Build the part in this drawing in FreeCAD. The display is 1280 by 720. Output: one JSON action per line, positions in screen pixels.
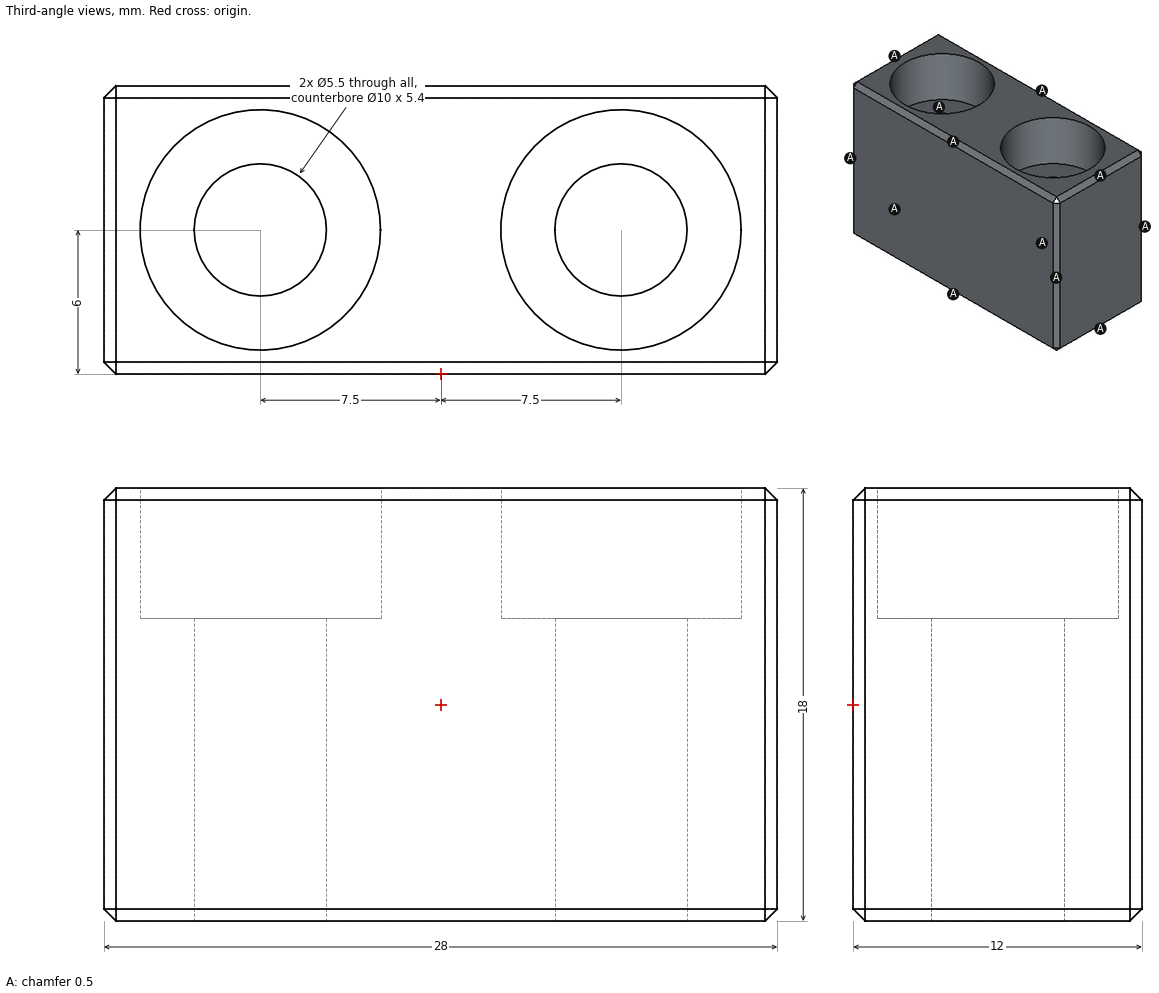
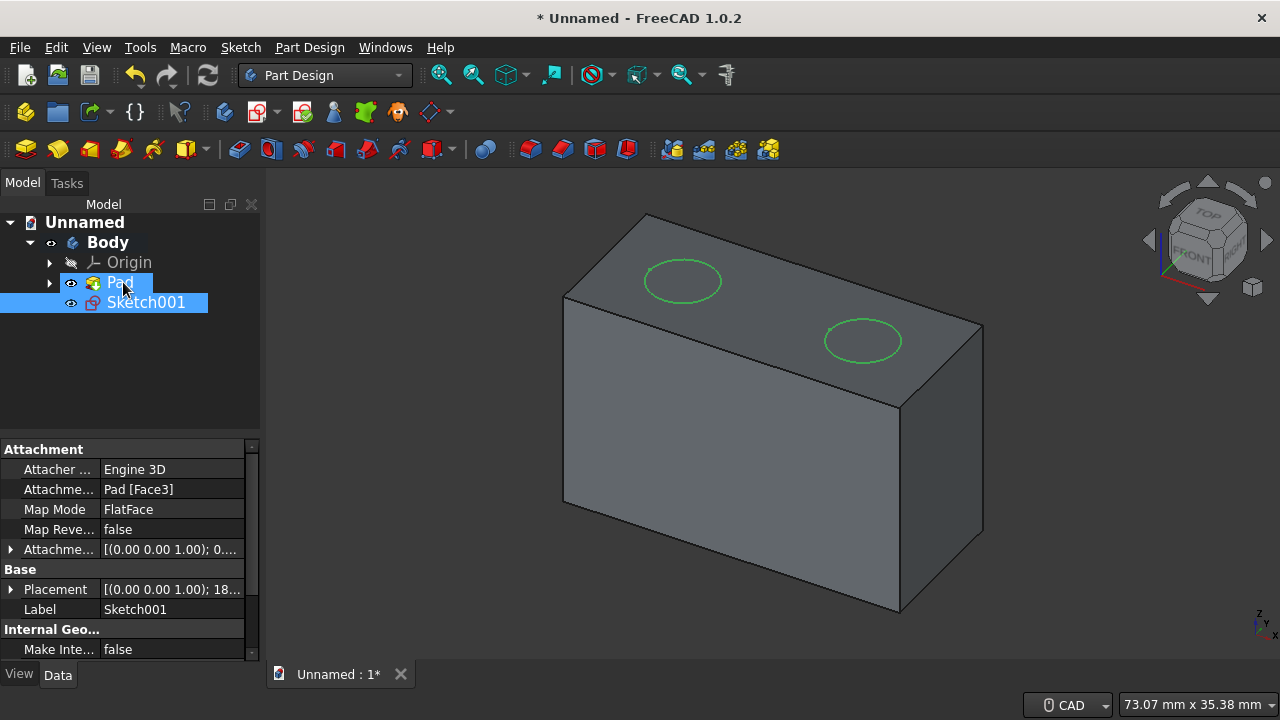
{"action": "left_click", "coordinate": [272, 150]}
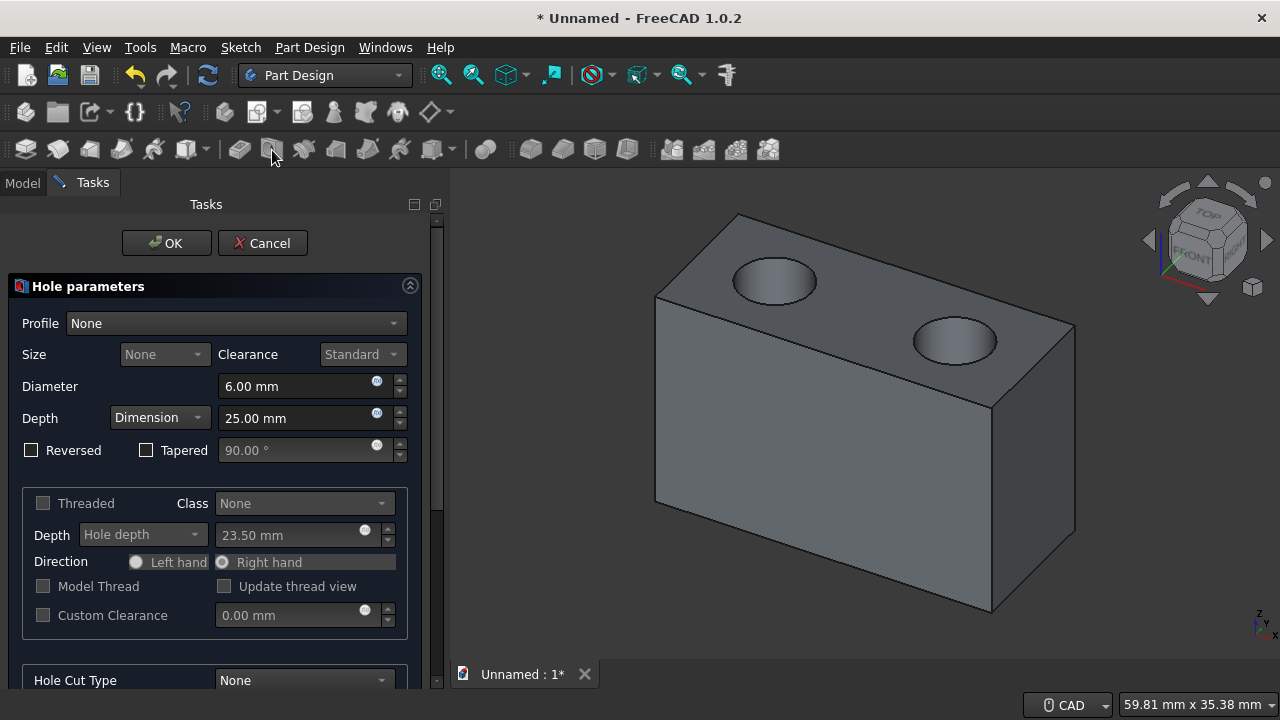
{"action": "triple_click", "coordinate": [305, 386]}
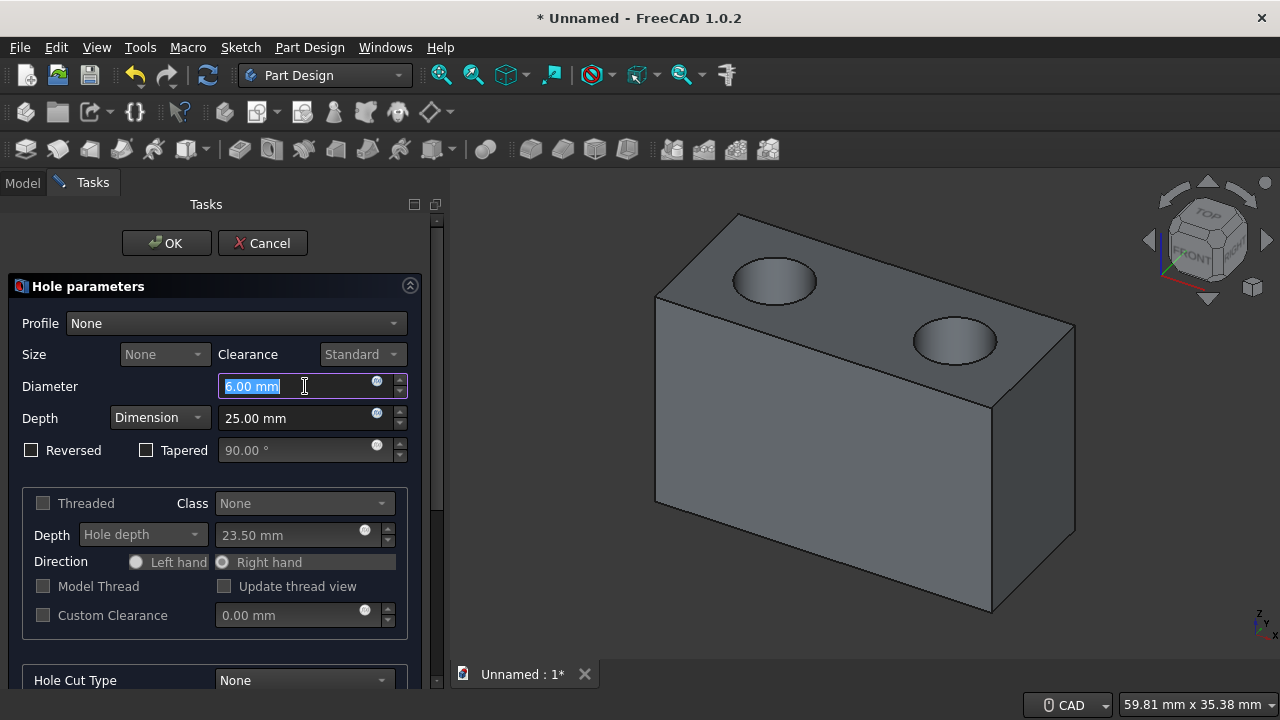
{"action": "type", "text": "5.5"}
{"action": "key", "text": "Tab"}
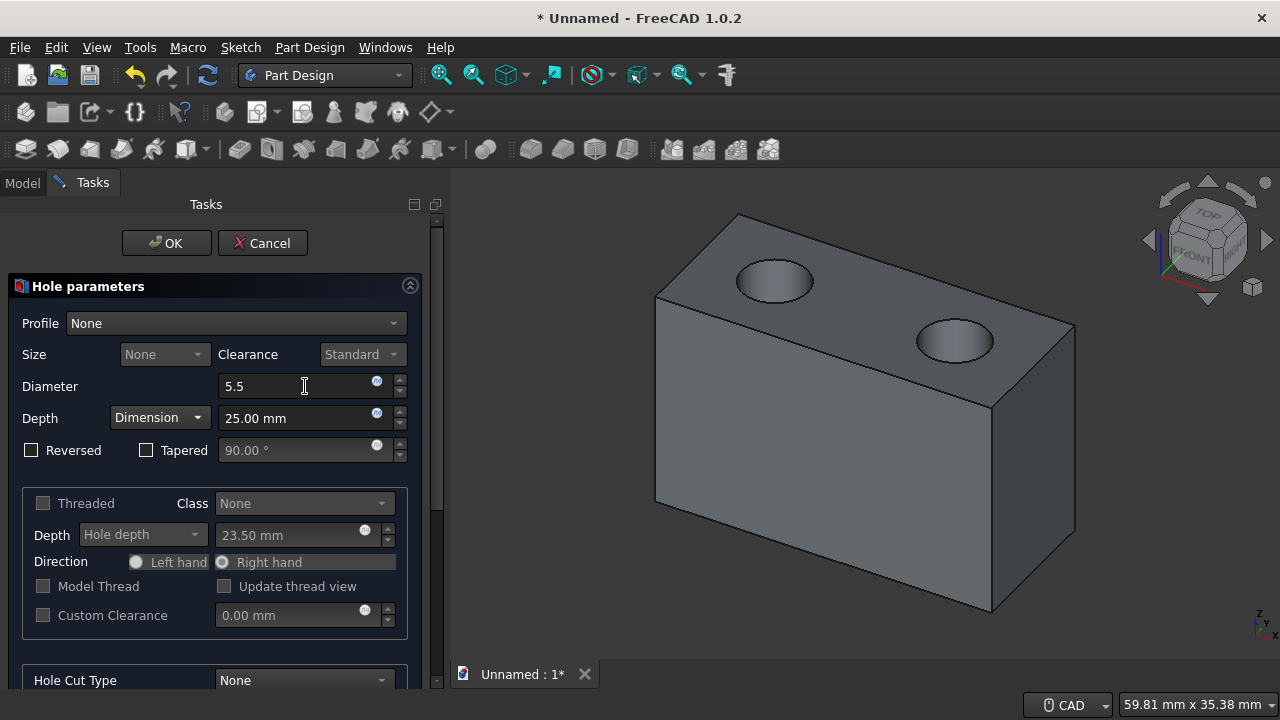
{"action": "left_click", "coordinate": [161, 418]}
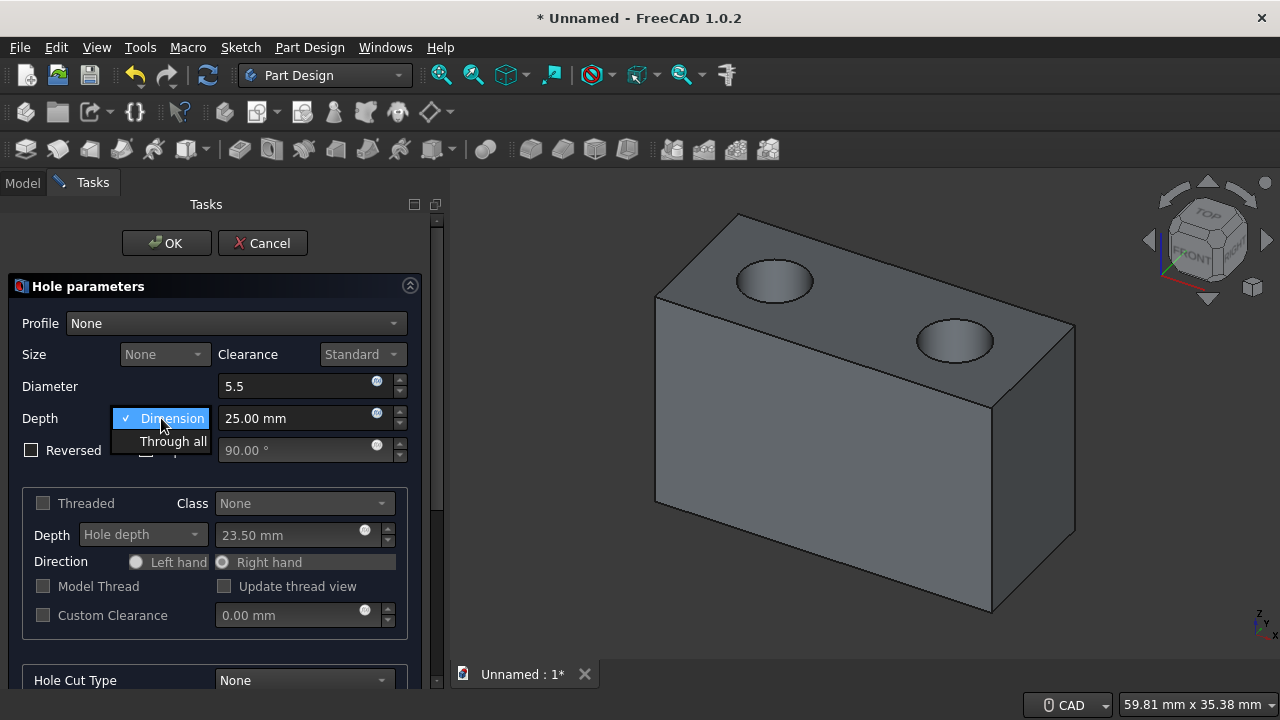
{"action": "left_click", "coordinate": [160, 442]}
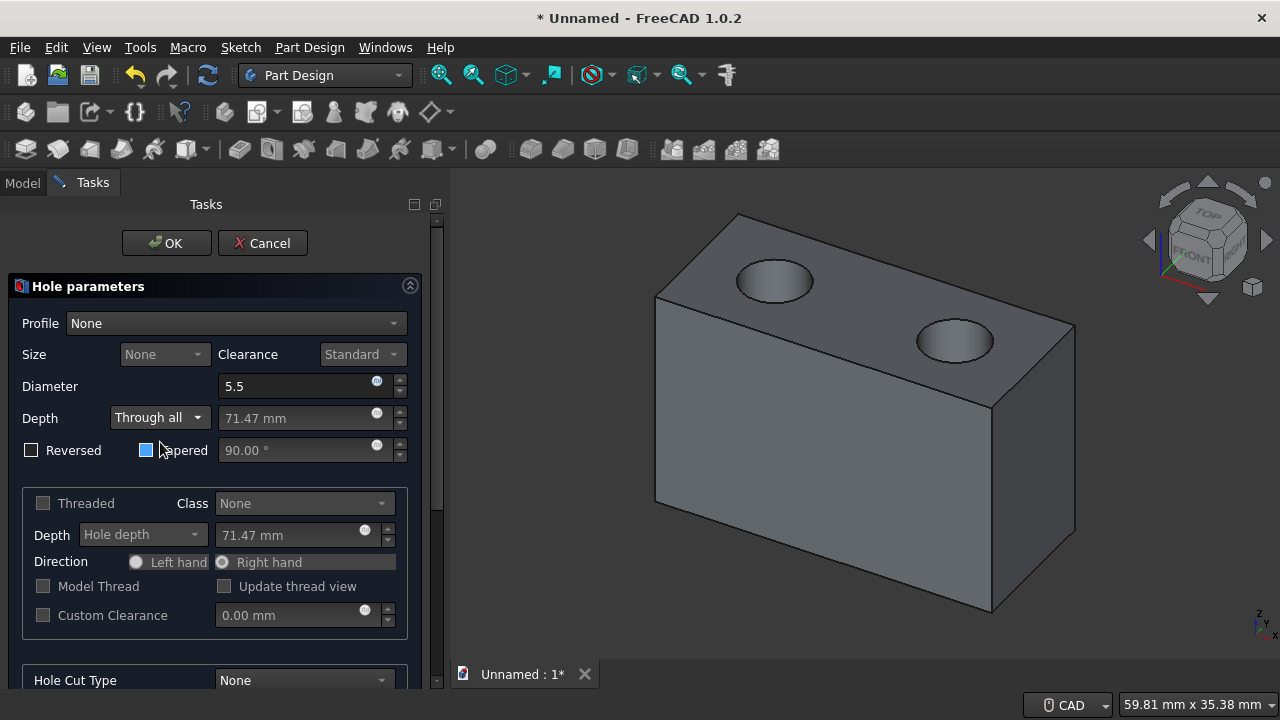
{"action": "scroll", "coordinate": [437, 451], "scroll_direction": "down", "scroll_amount": 2}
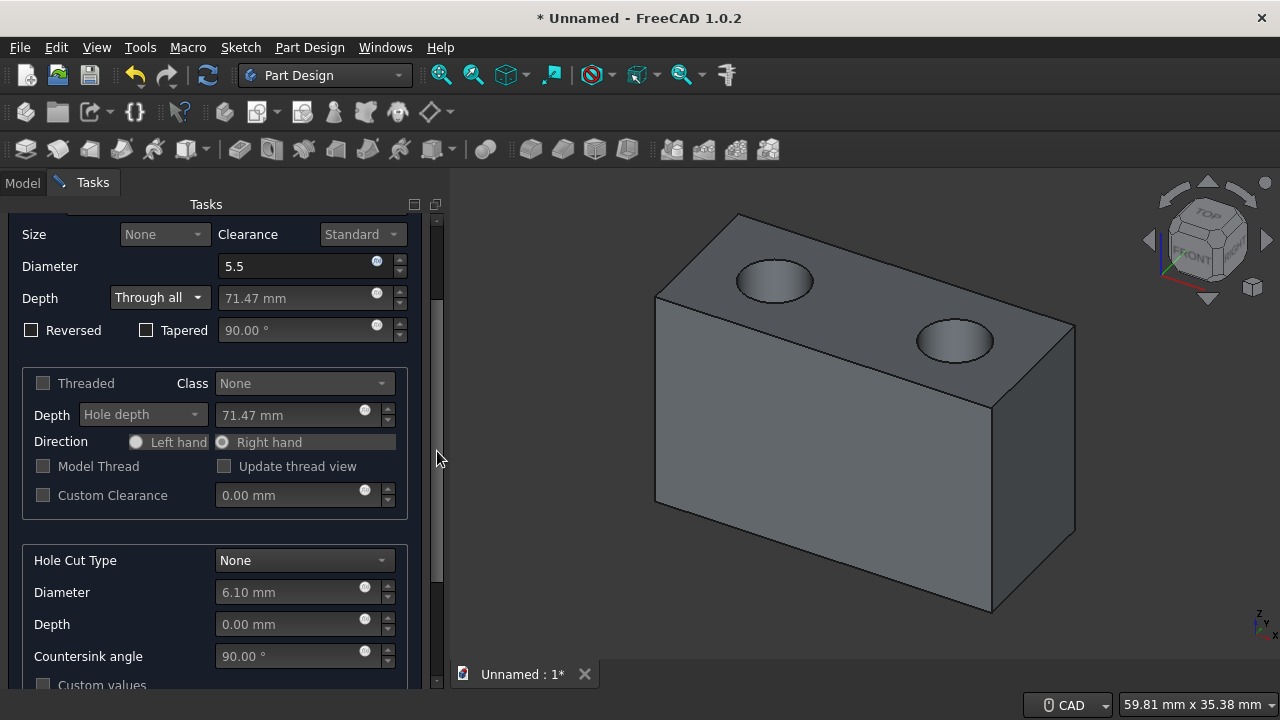
{"action": "left_click", "coordinate": [306, 560]}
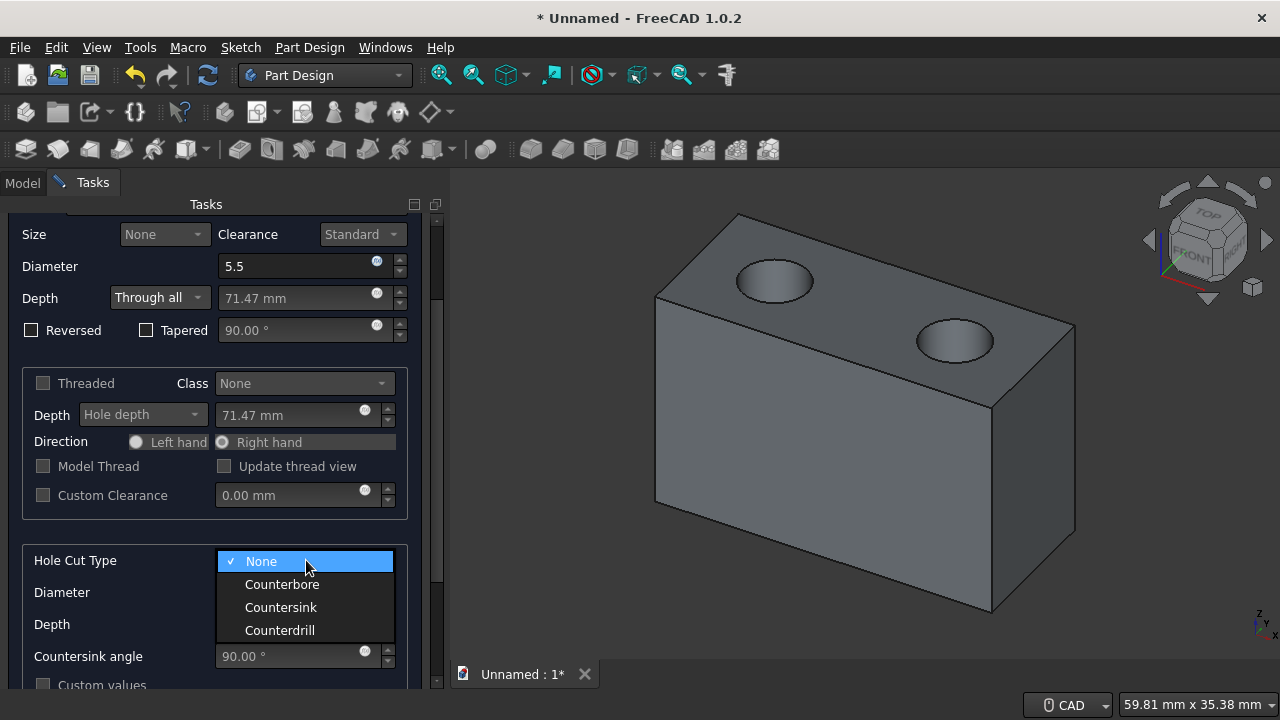
{"action": "left_click", "coordinate": [304, 584]}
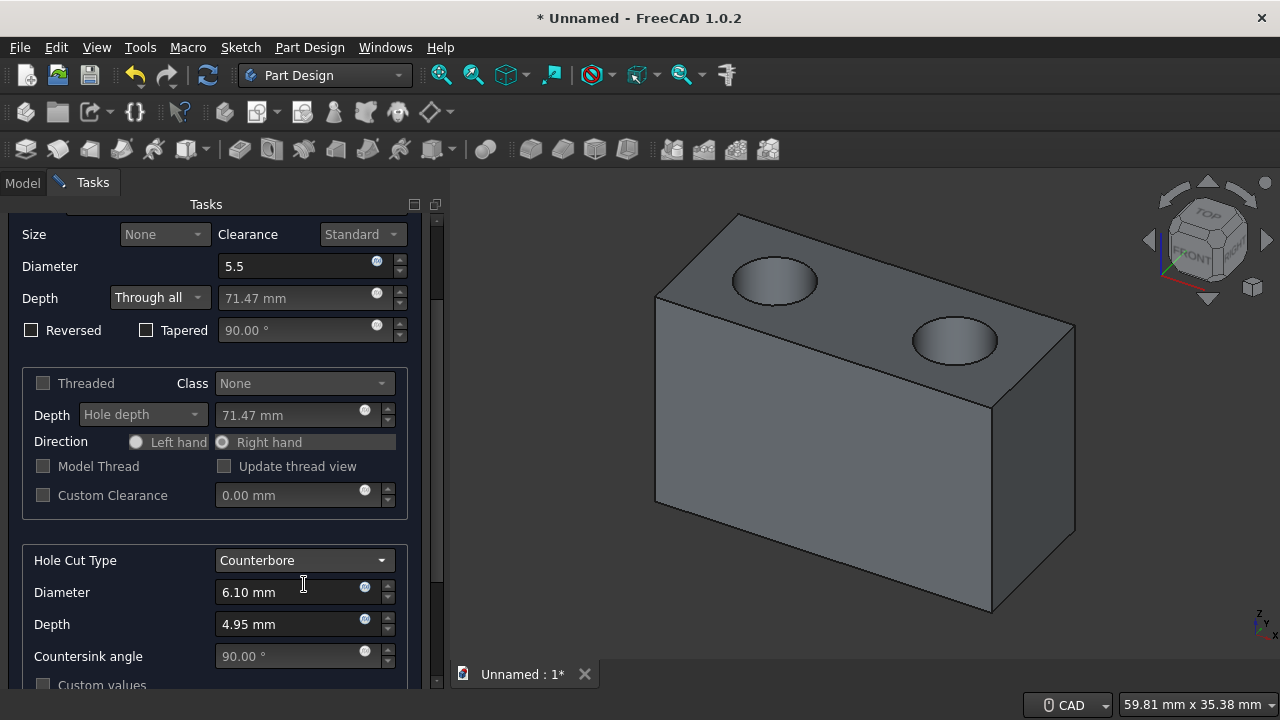
{"action": "triple_click", "coordinate": [298, 592]}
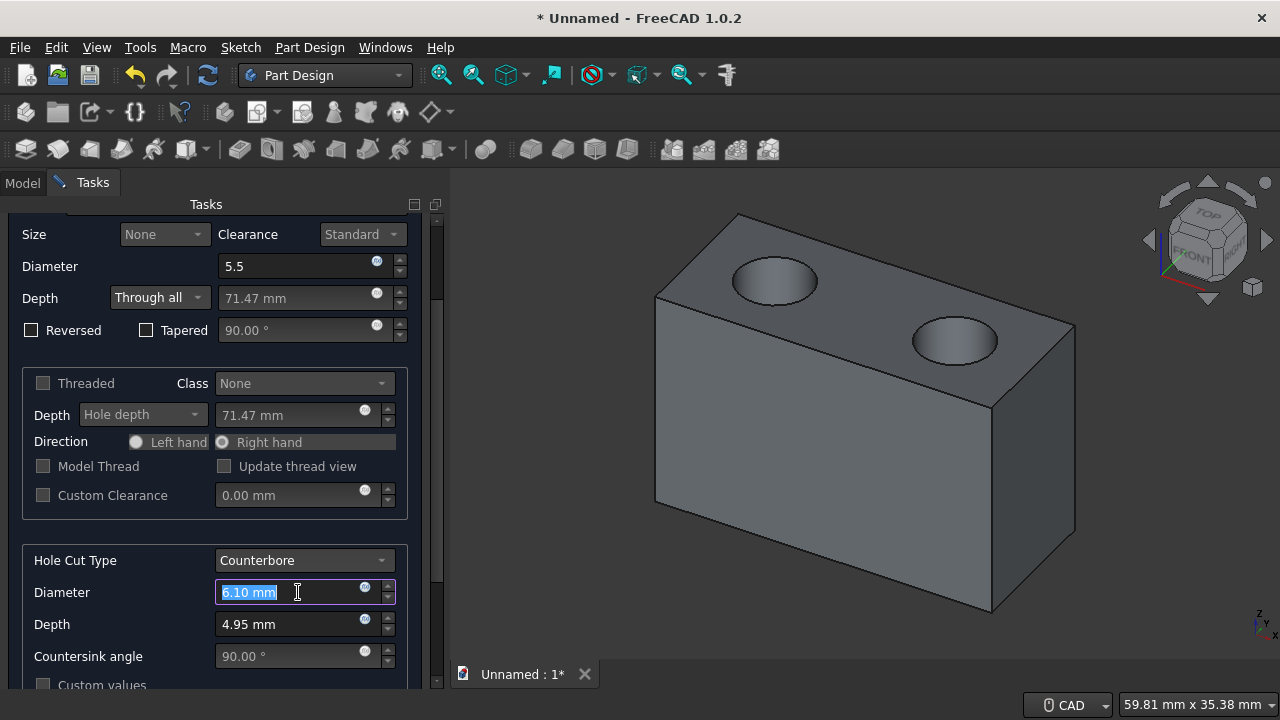
{"action": "type", "text": "10"}
{"action": "key", "text": "Tab"}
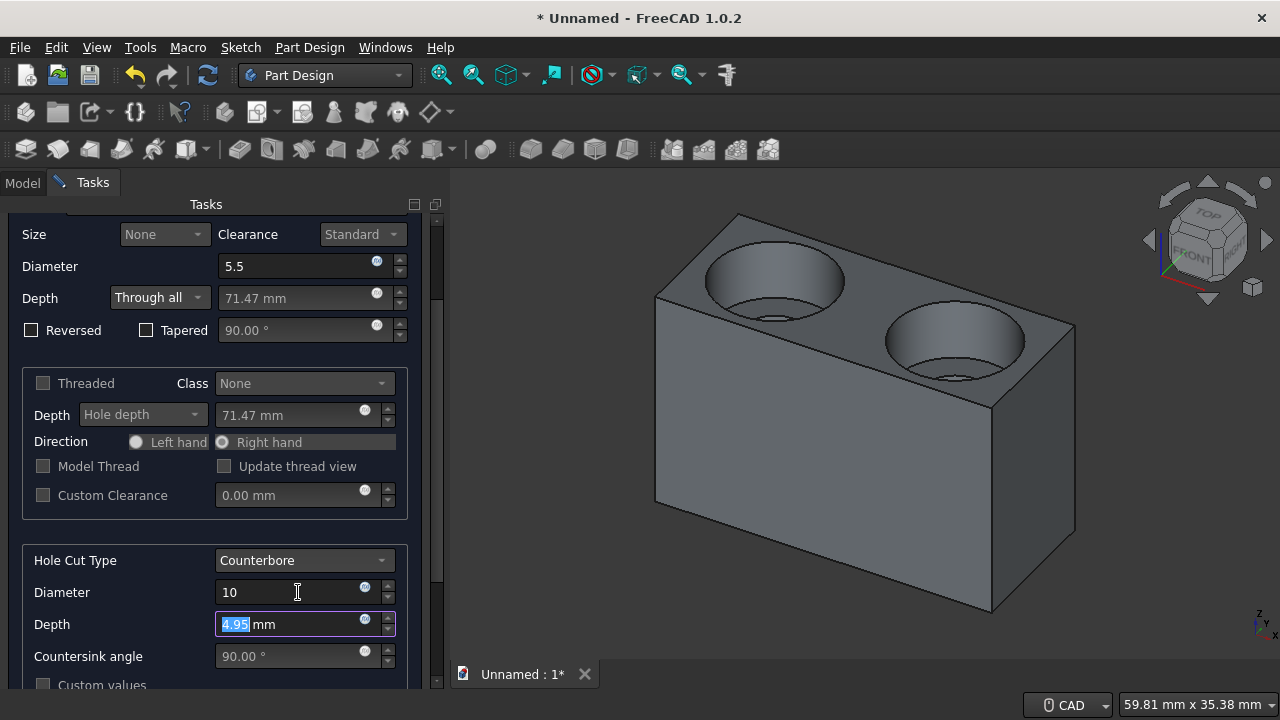
{"action": "type", "text": "5.4"}
{"action": "key", "text": "Tab"}